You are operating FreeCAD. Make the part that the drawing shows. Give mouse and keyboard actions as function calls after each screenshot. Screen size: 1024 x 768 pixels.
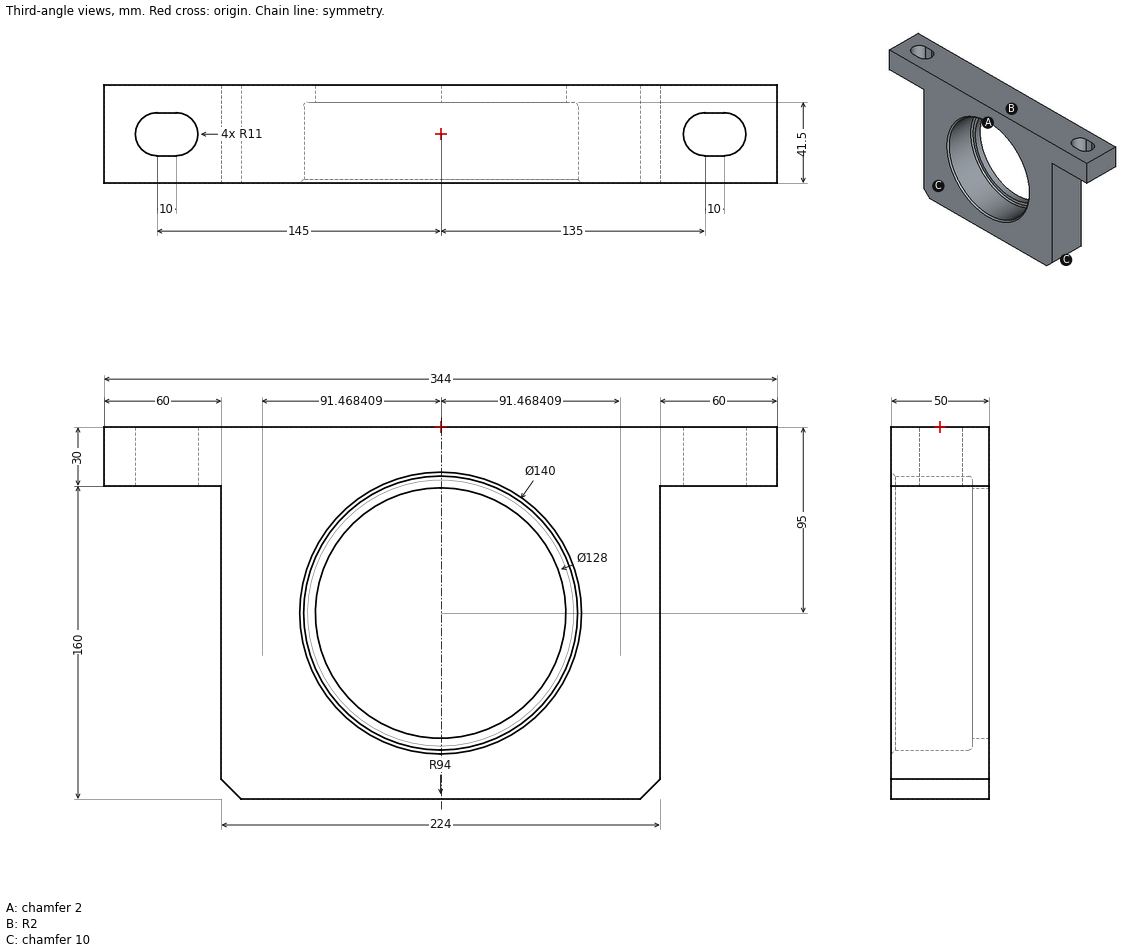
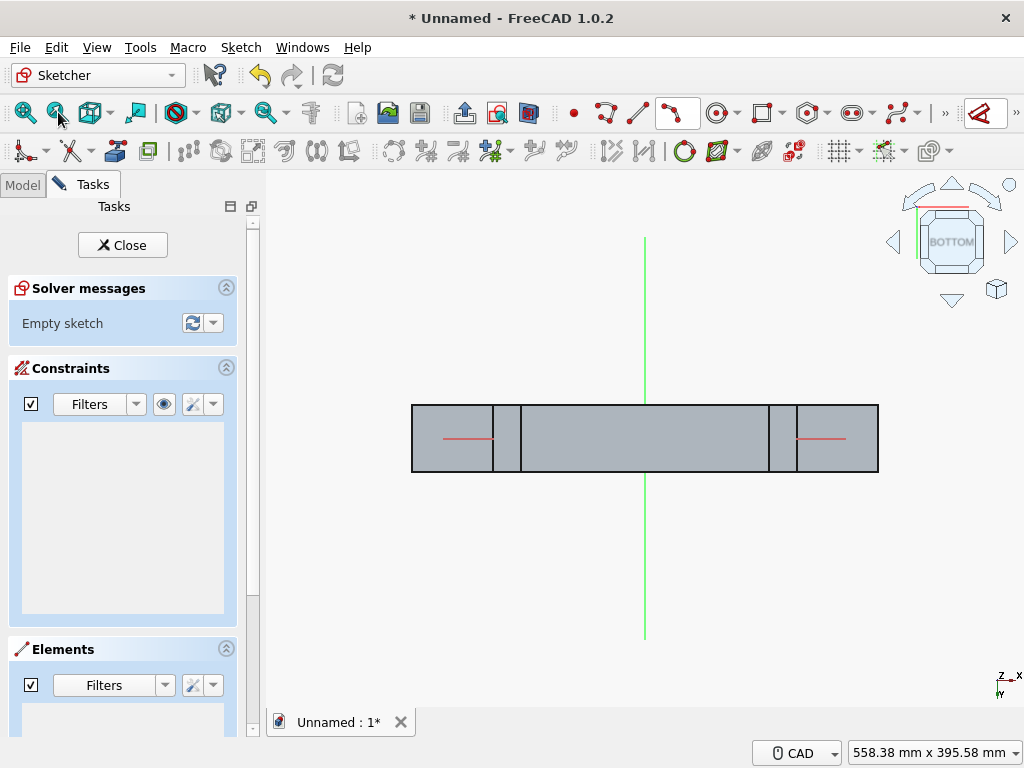
scroll(294, 439, down, 1)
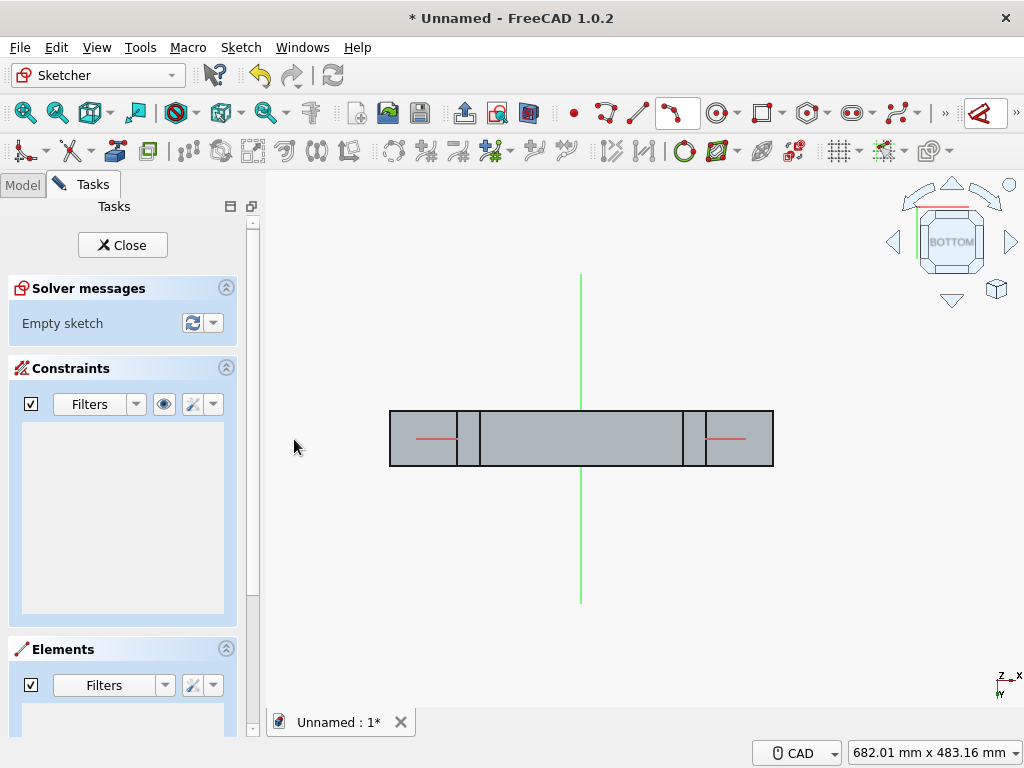
click(852, 114)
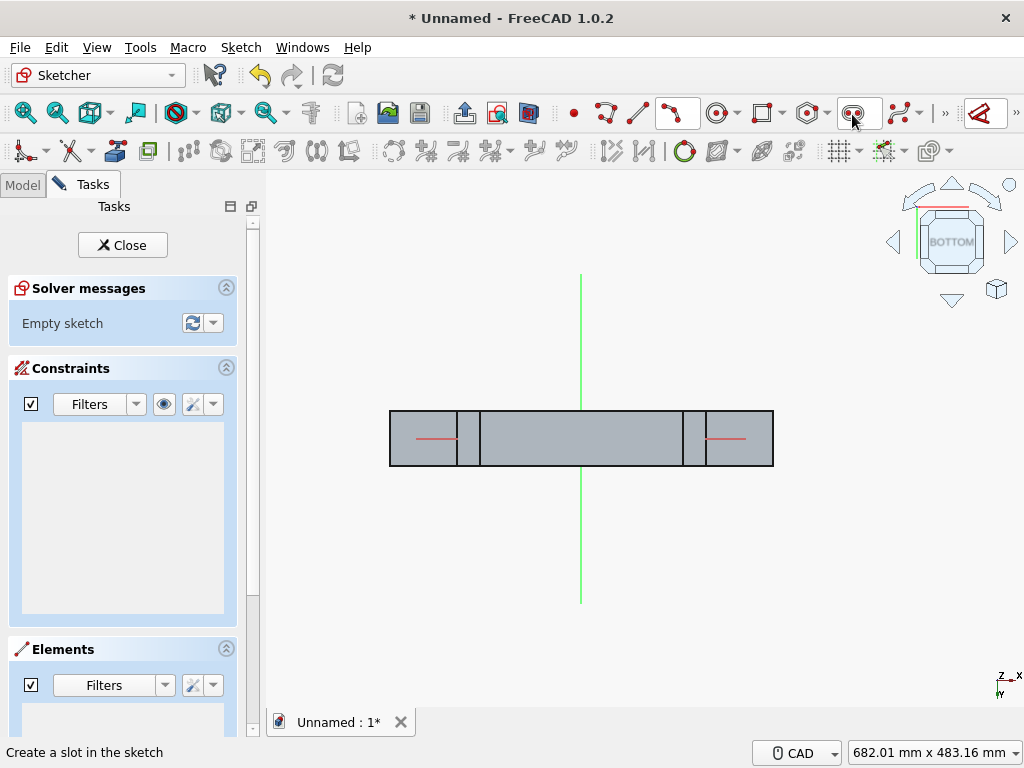
scroll(420, 439, up, 4)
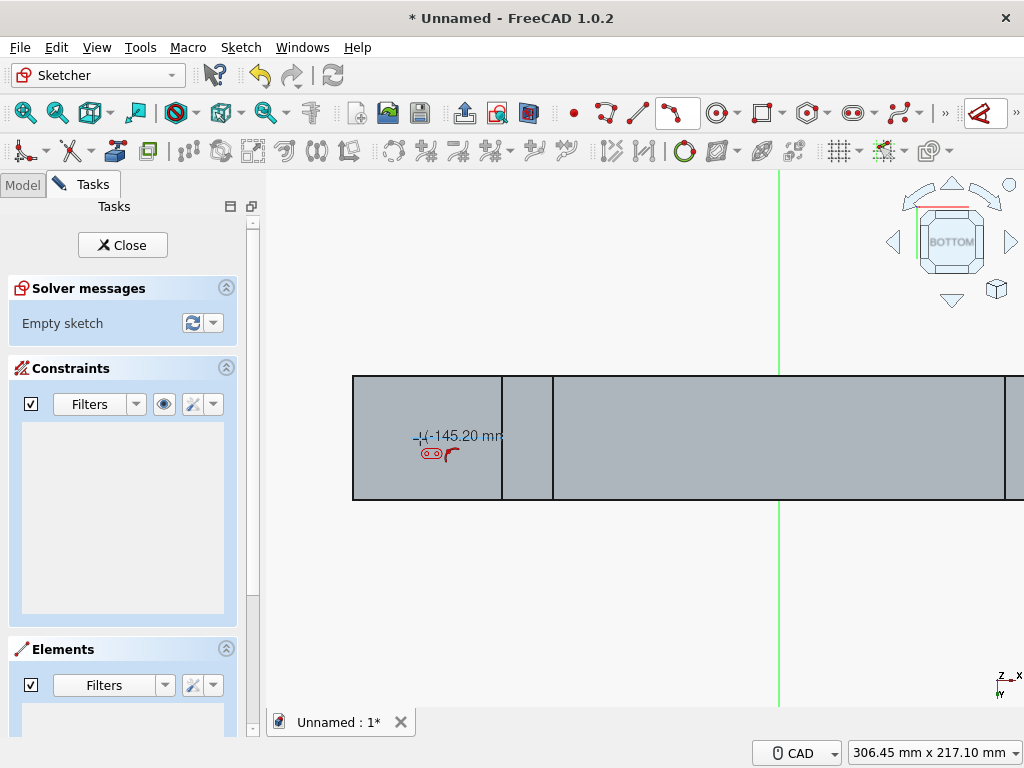
click(420, 438)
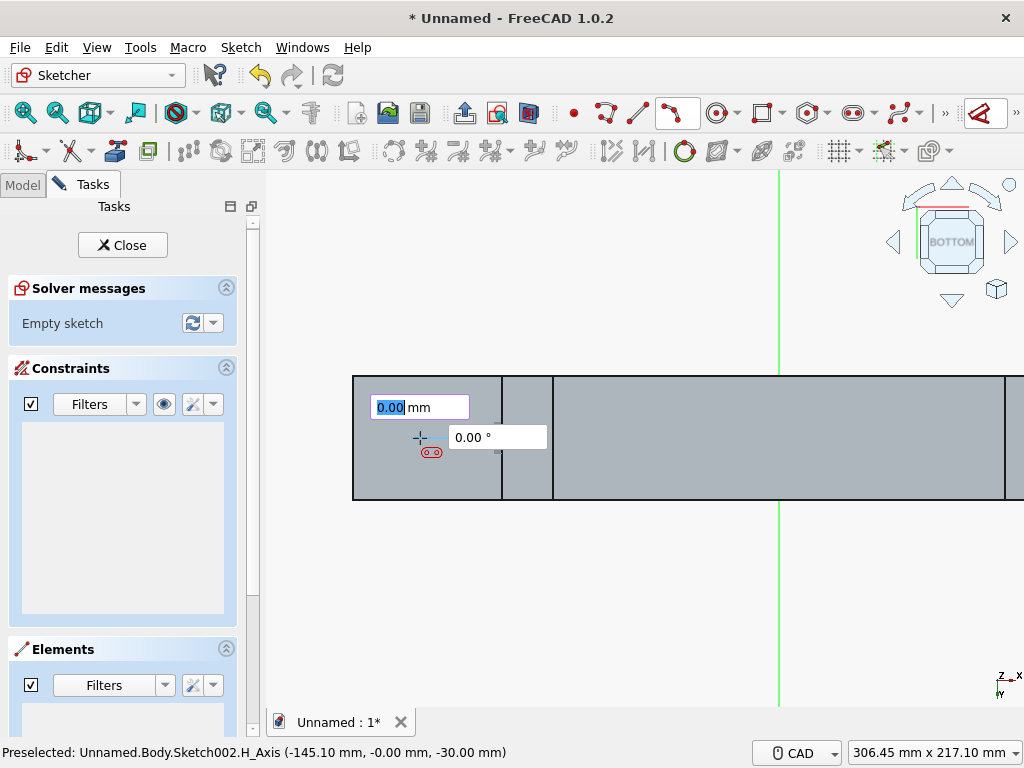
click(445, 429)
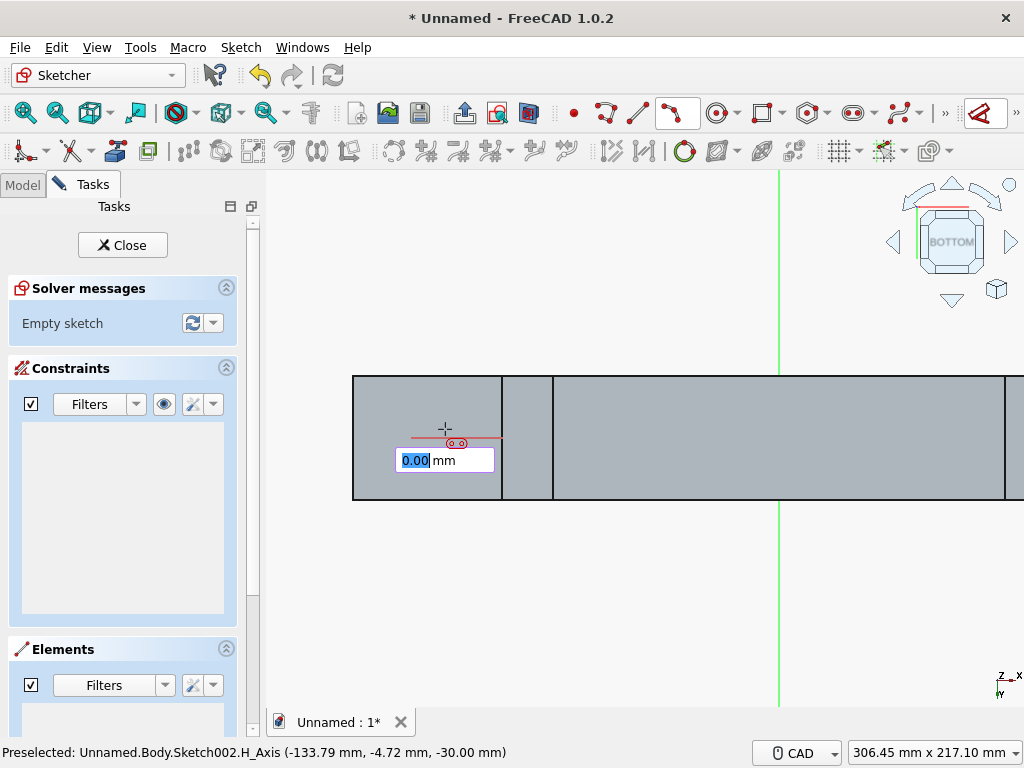
click(433, 465)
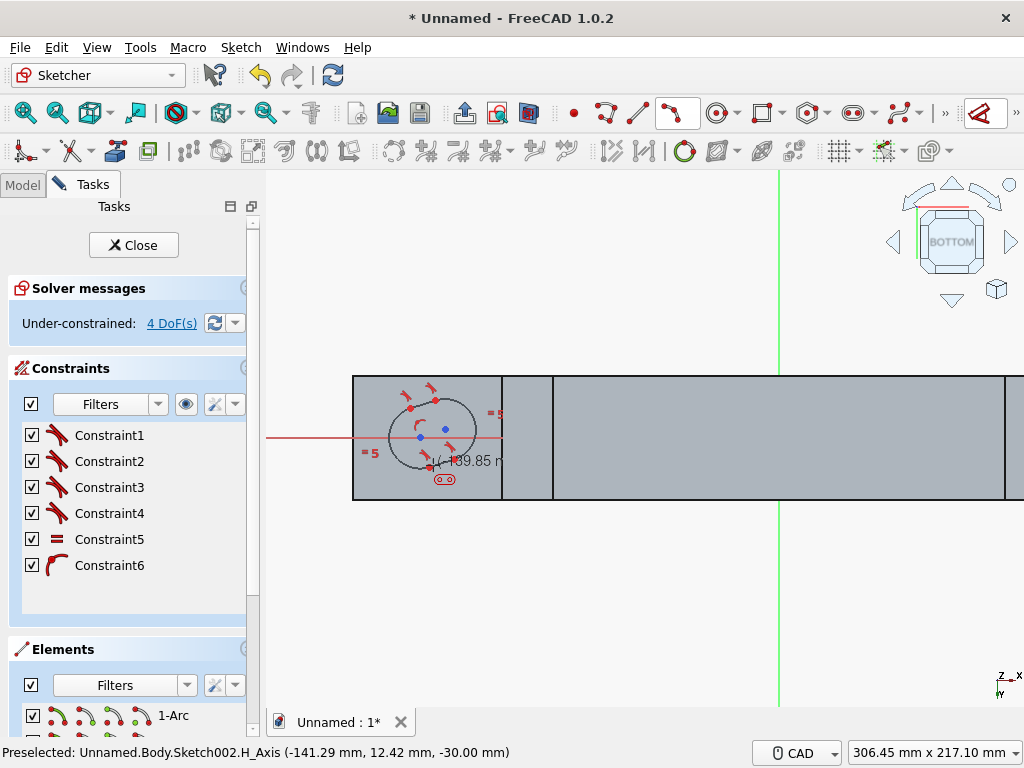
scroll(330, 440, down, 3)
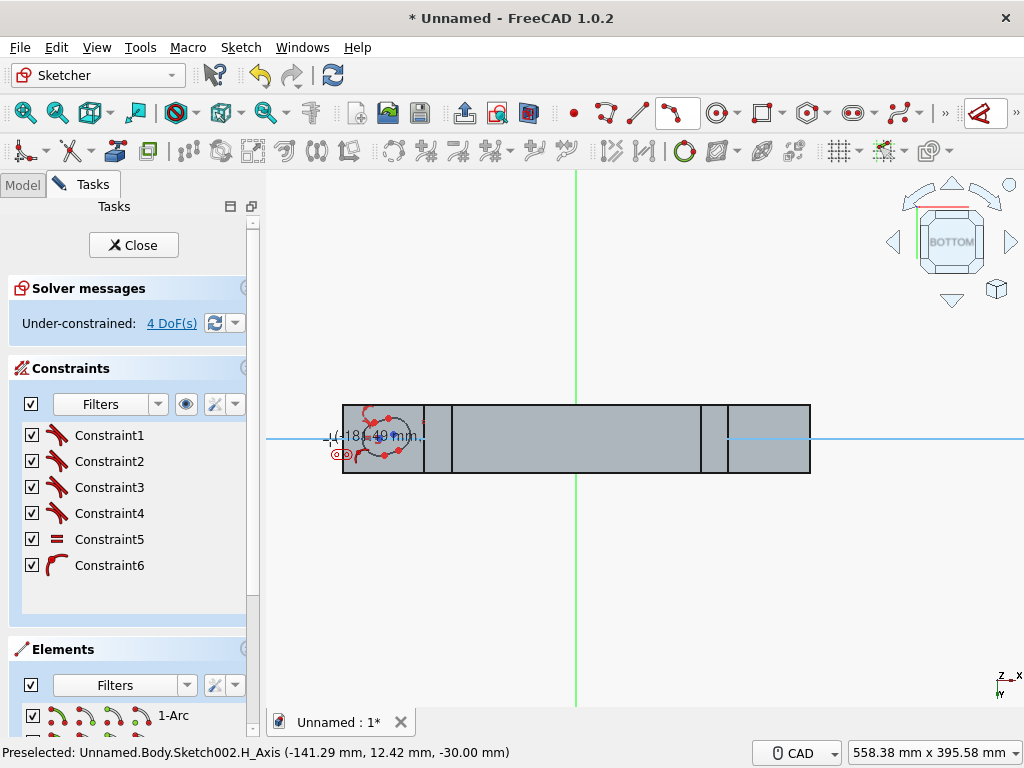
scroll(760, 439, up, 3)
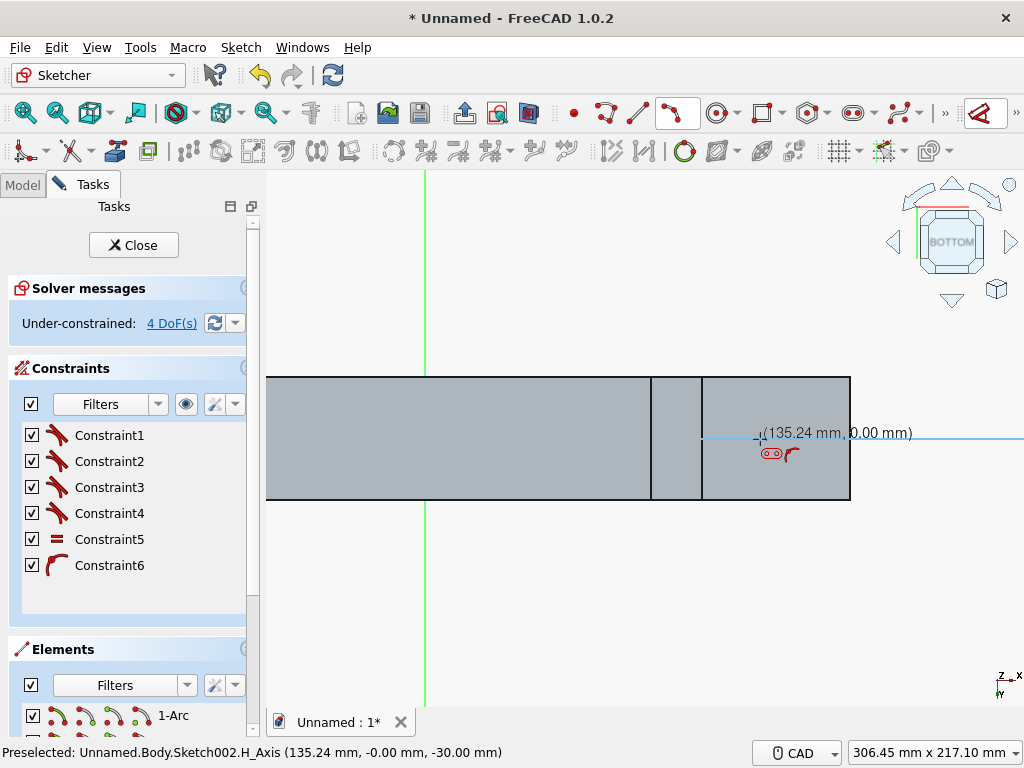
click(759, 438)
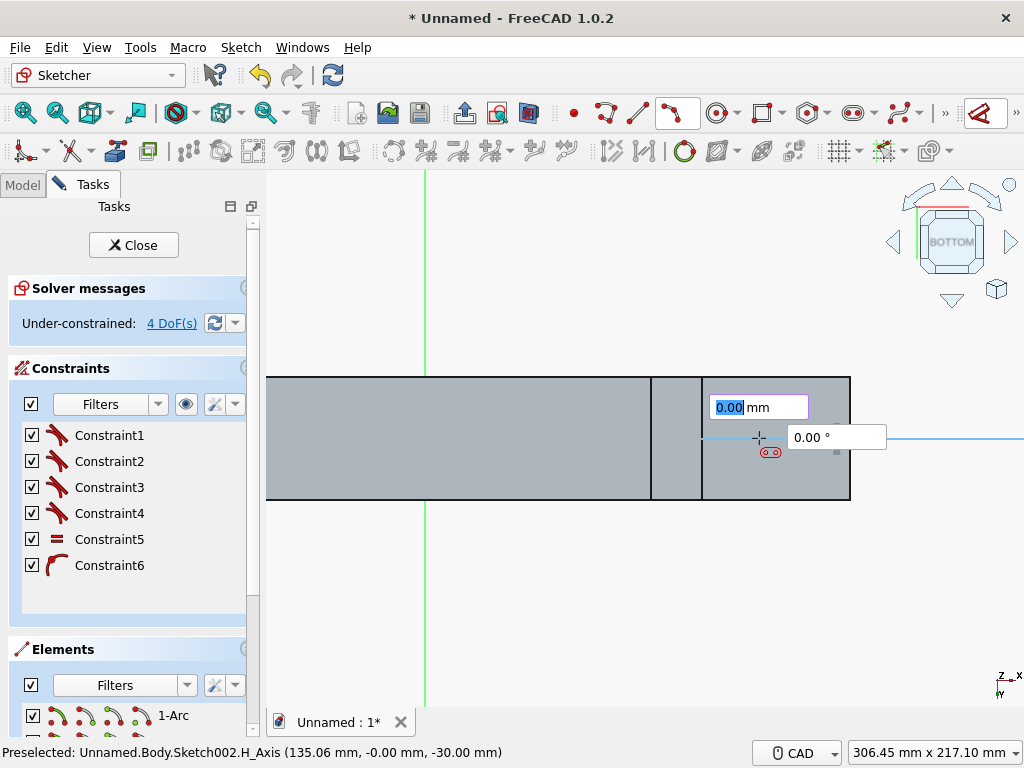
click(784, 429)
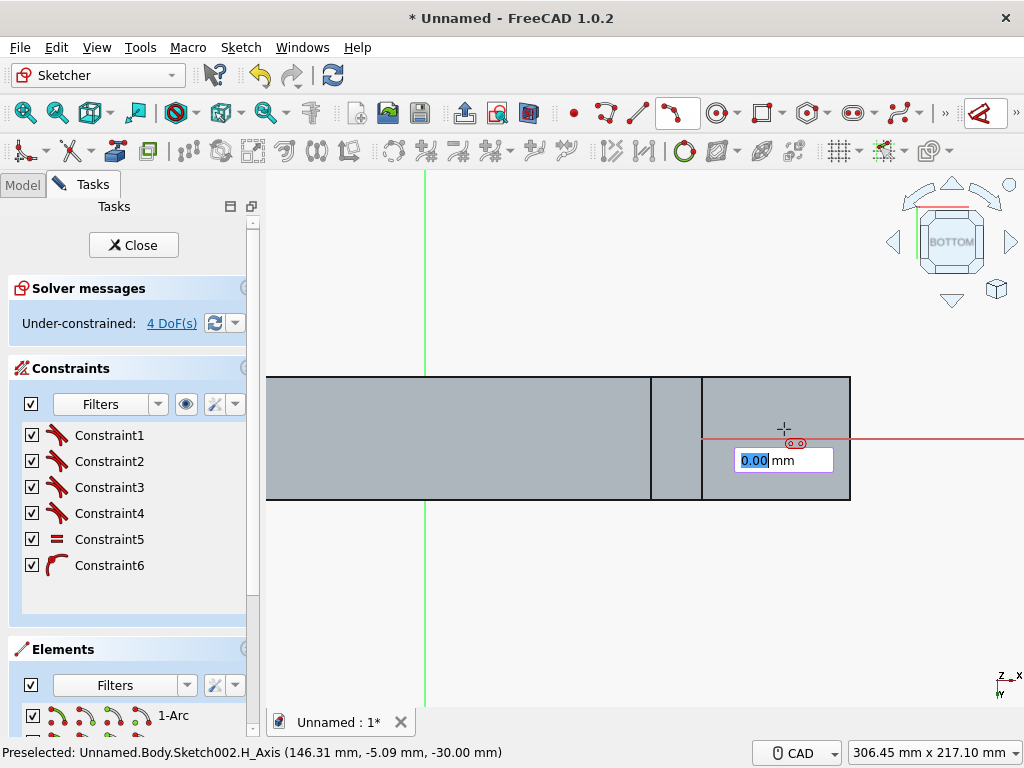
click(771, 466)
key(Escape)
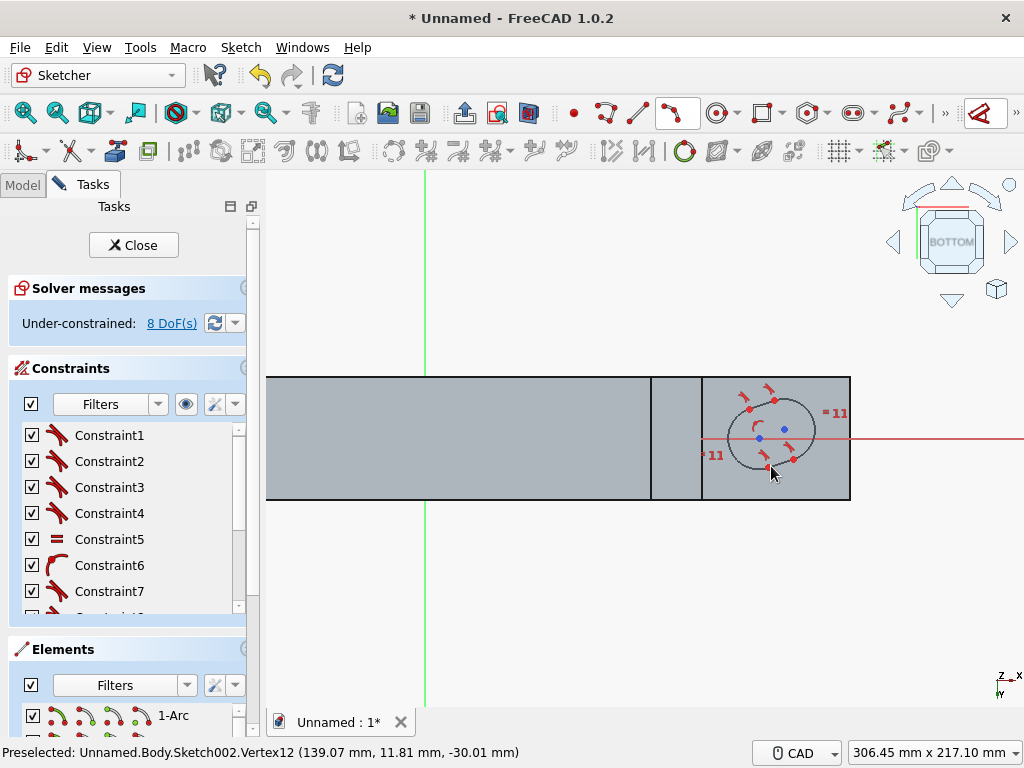
scroll(761, 439, down, 3)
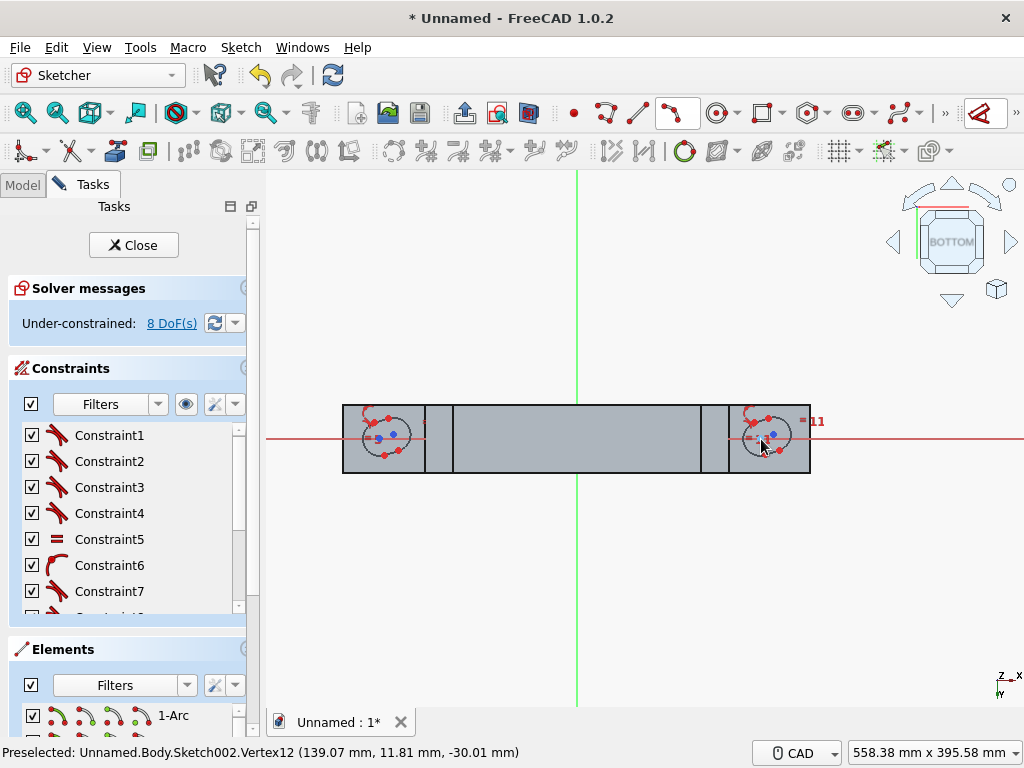
scroll(380, 421, up, 5)